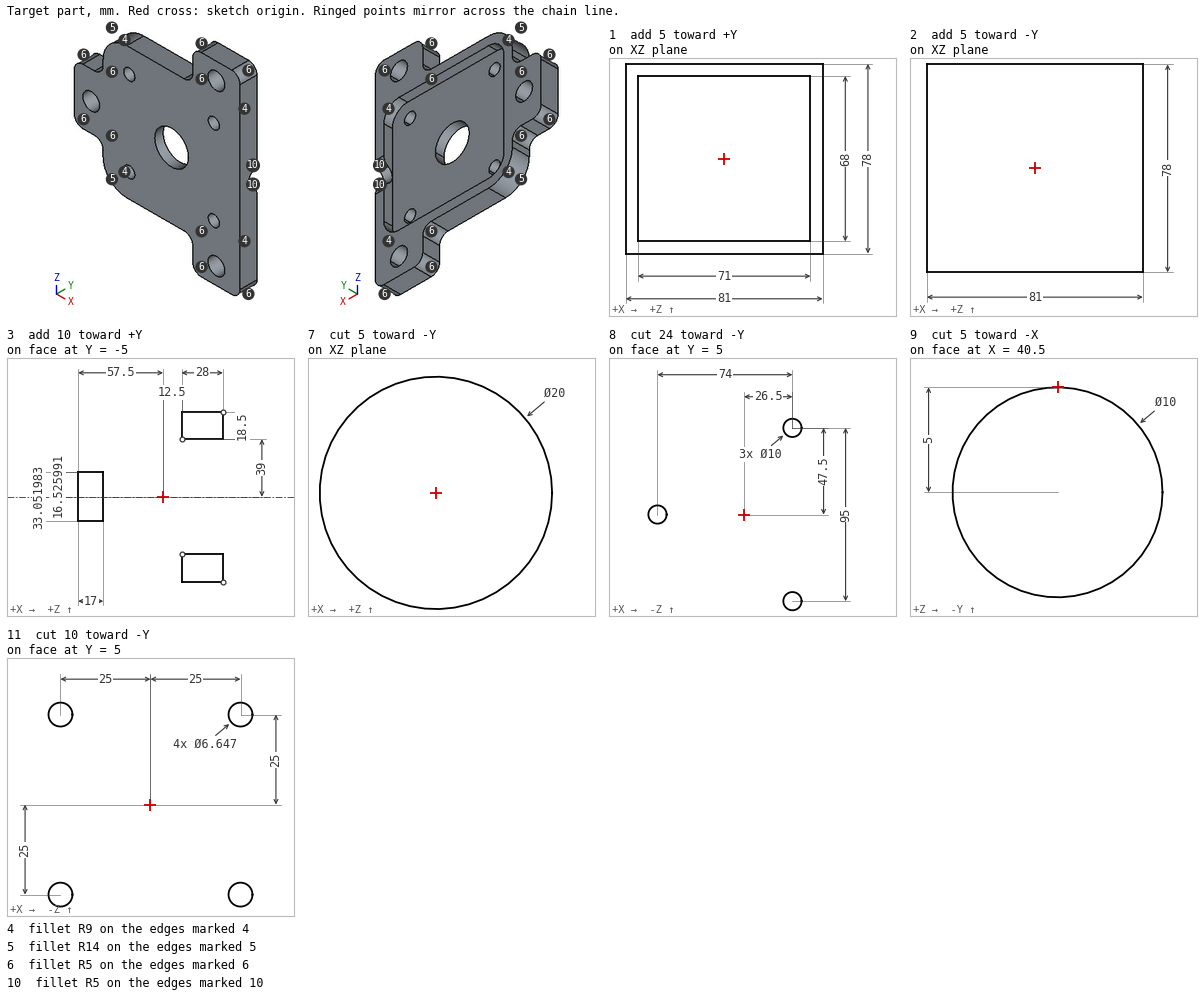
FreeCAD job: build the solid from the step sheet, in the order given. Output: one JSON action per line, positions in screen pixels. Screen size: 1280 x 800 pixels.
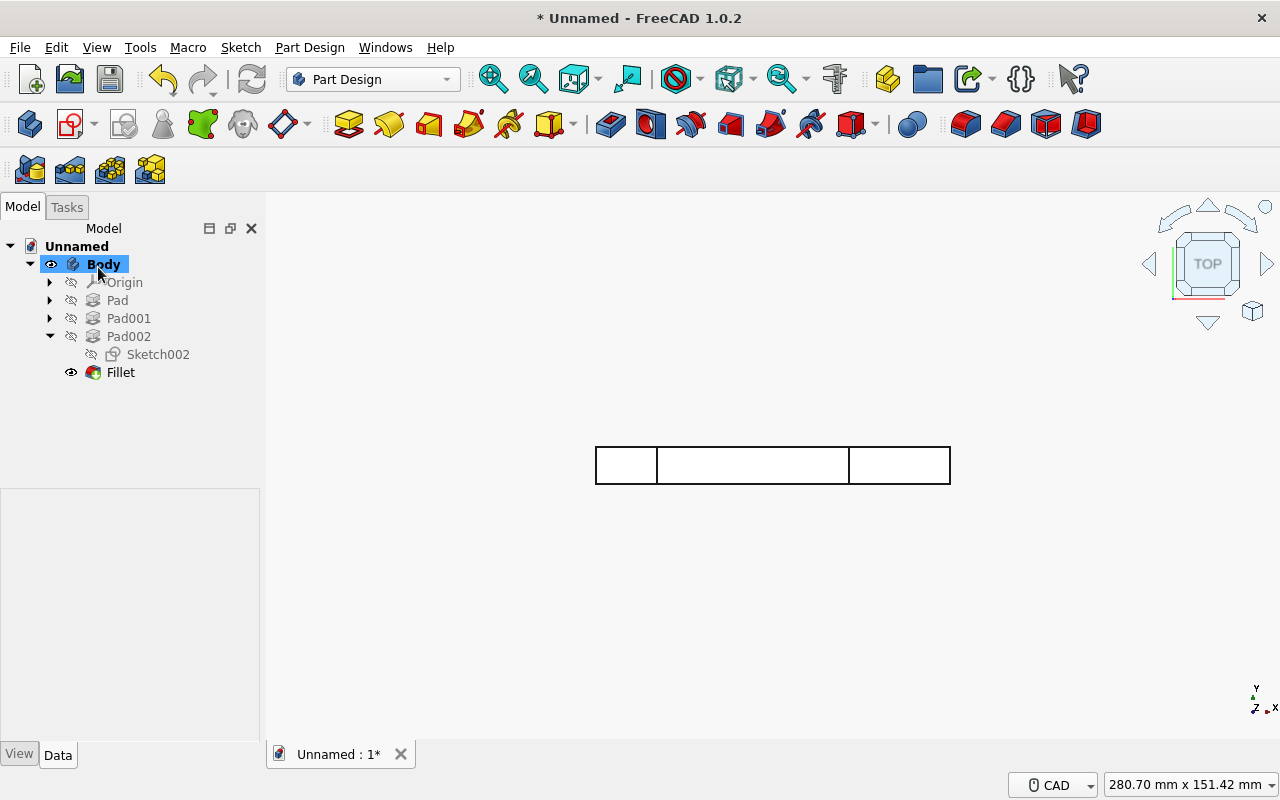
{"action": "key", "text": "v f"}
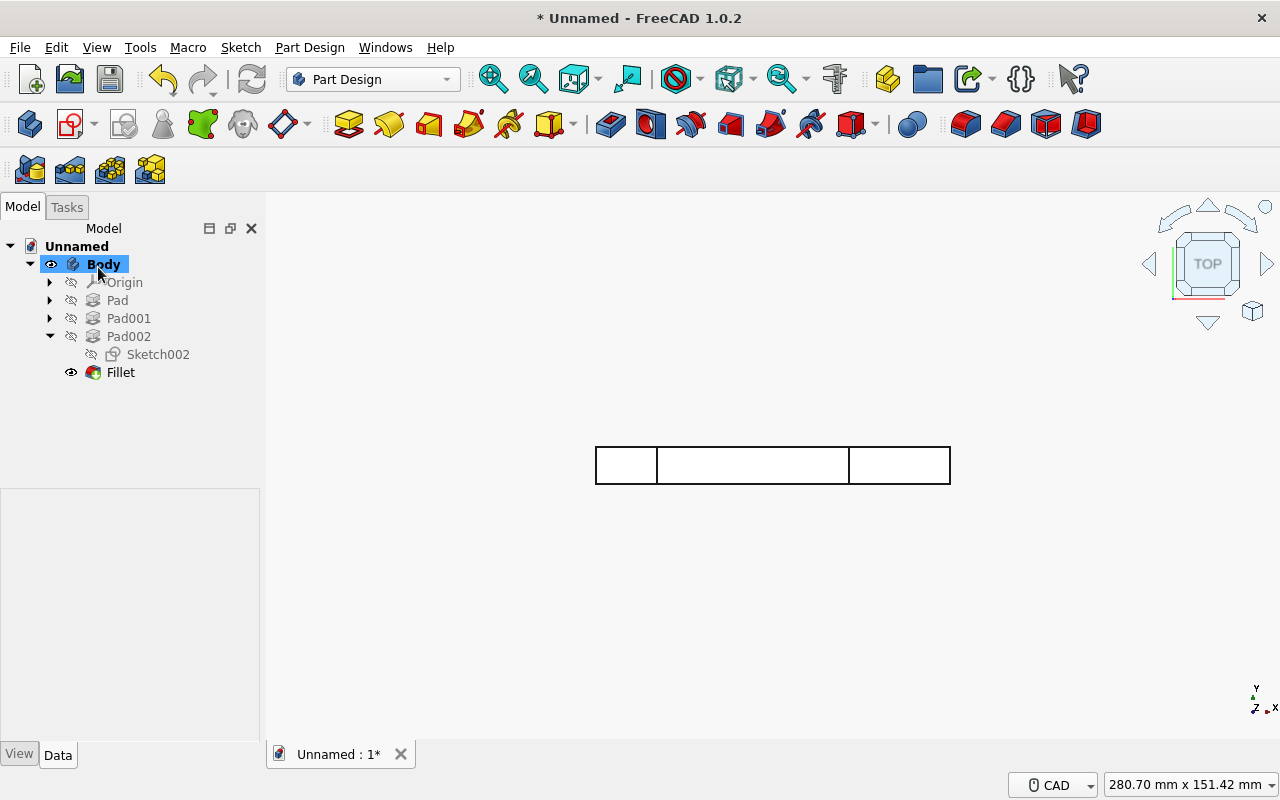
{"action": "left_click", "coordinate": [657, 464]}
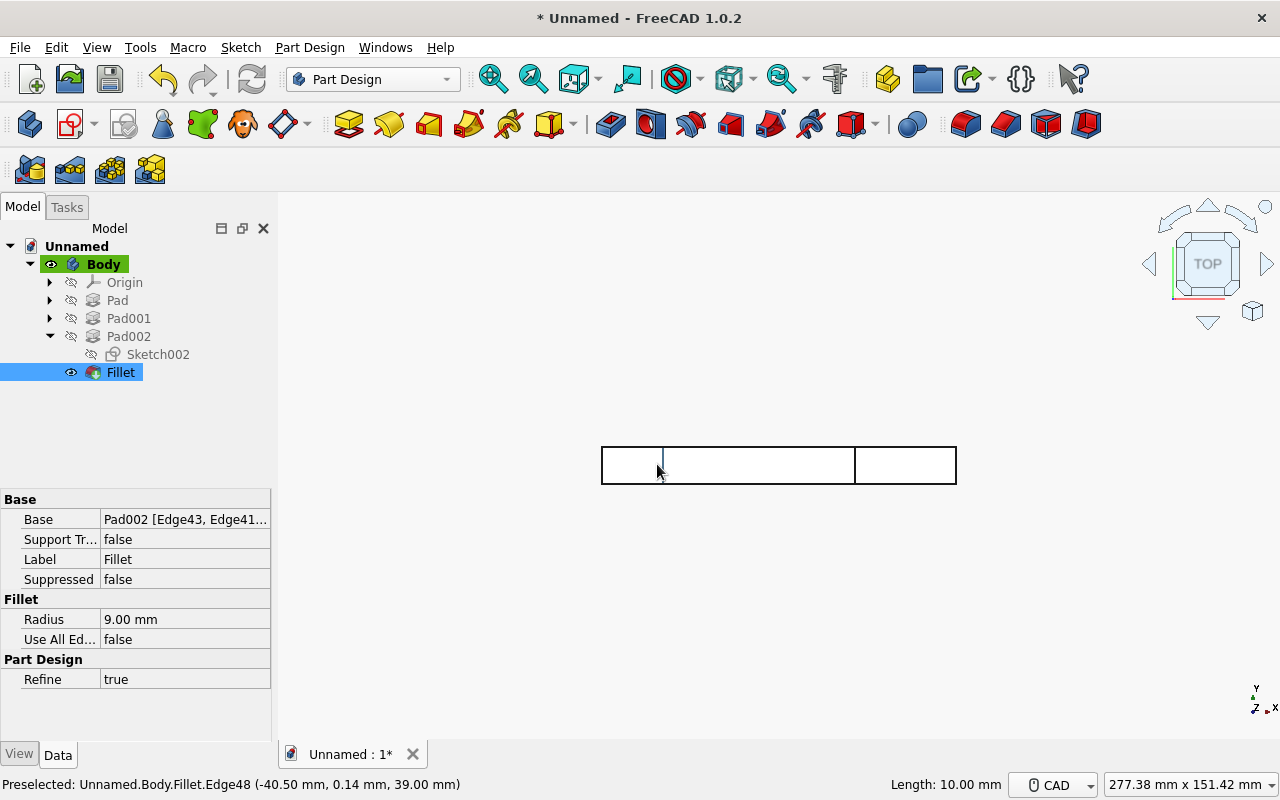
{"action": "key", "text": "0"}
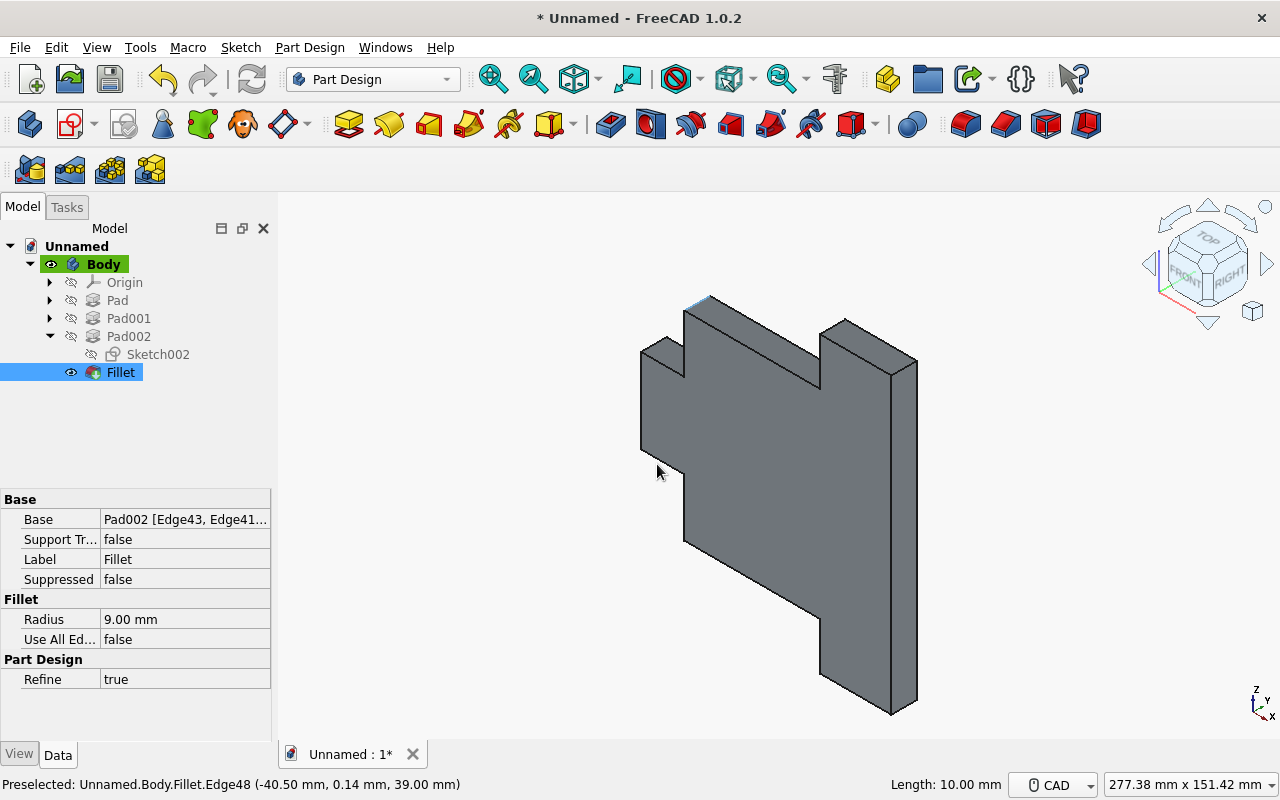
{"action": "key", "text": "1"}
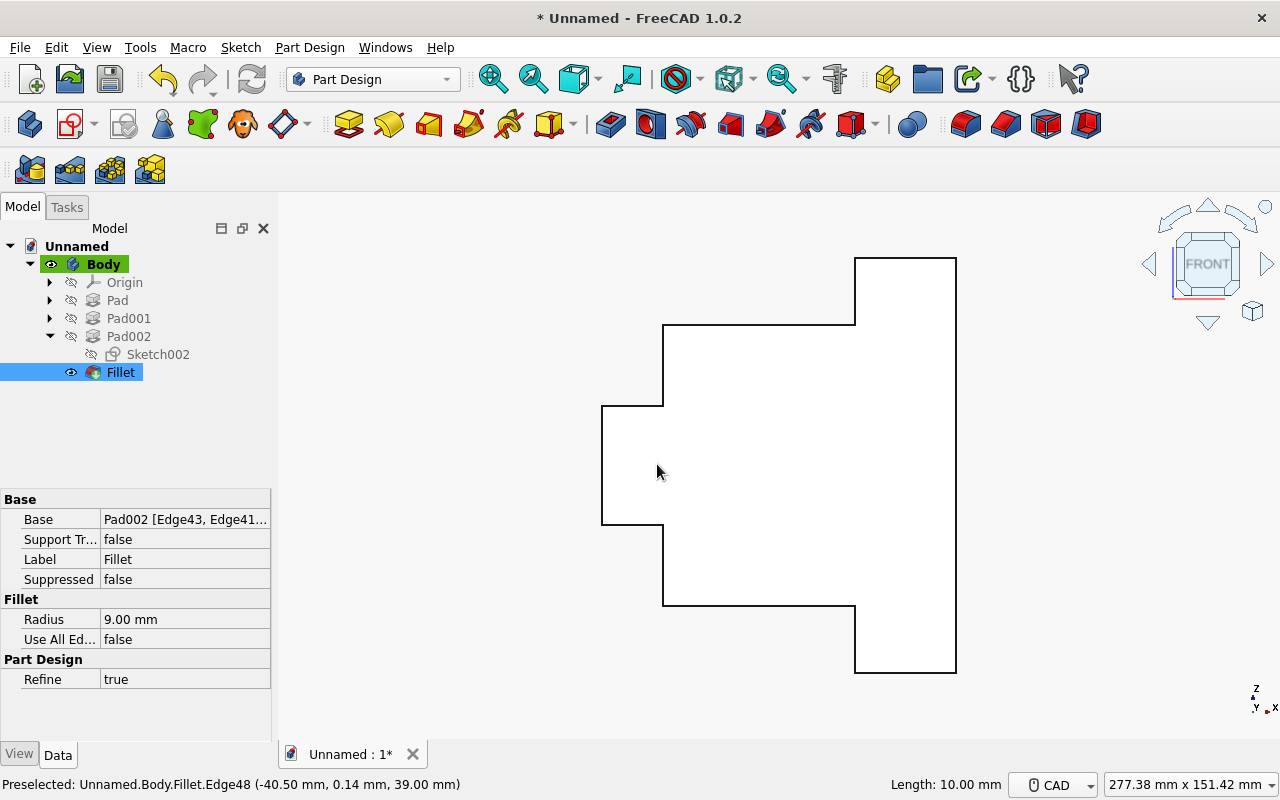
{"action": "key", "text": "3"}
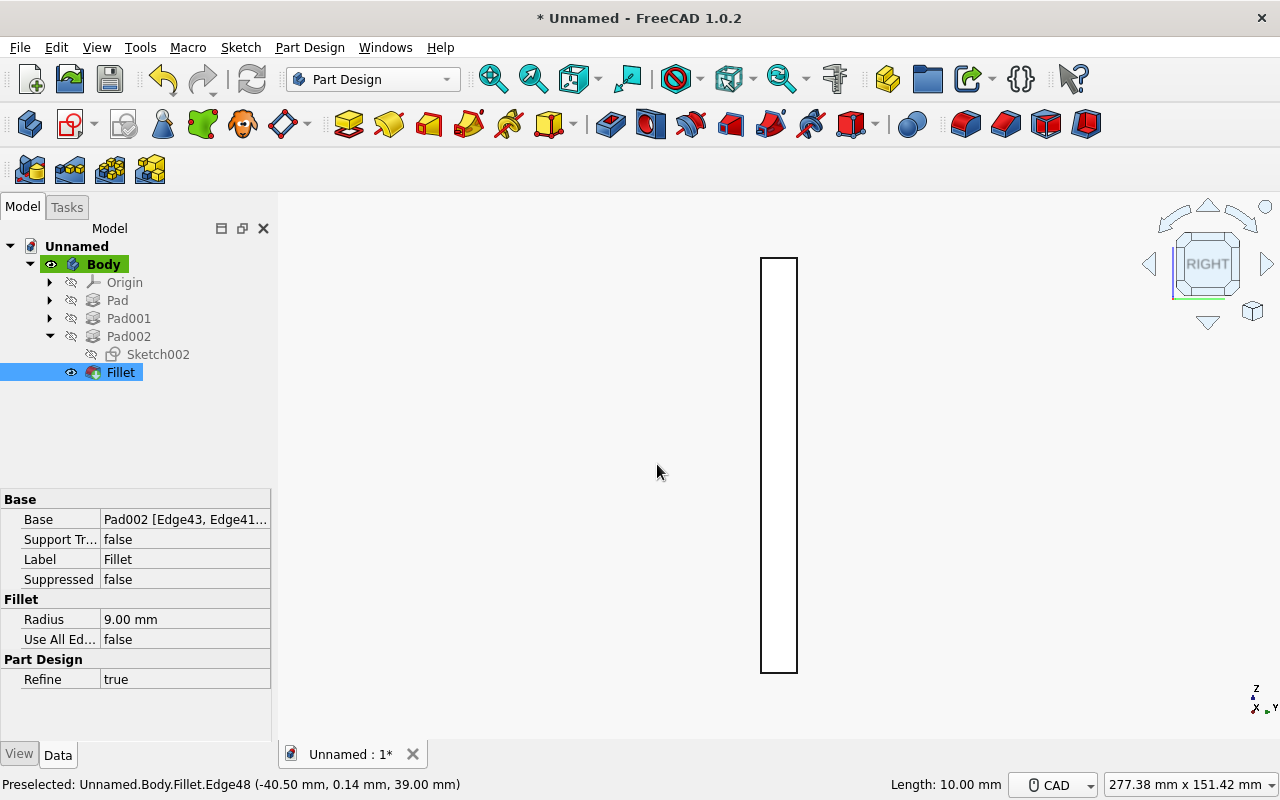
{"action": "key", "text": "5"}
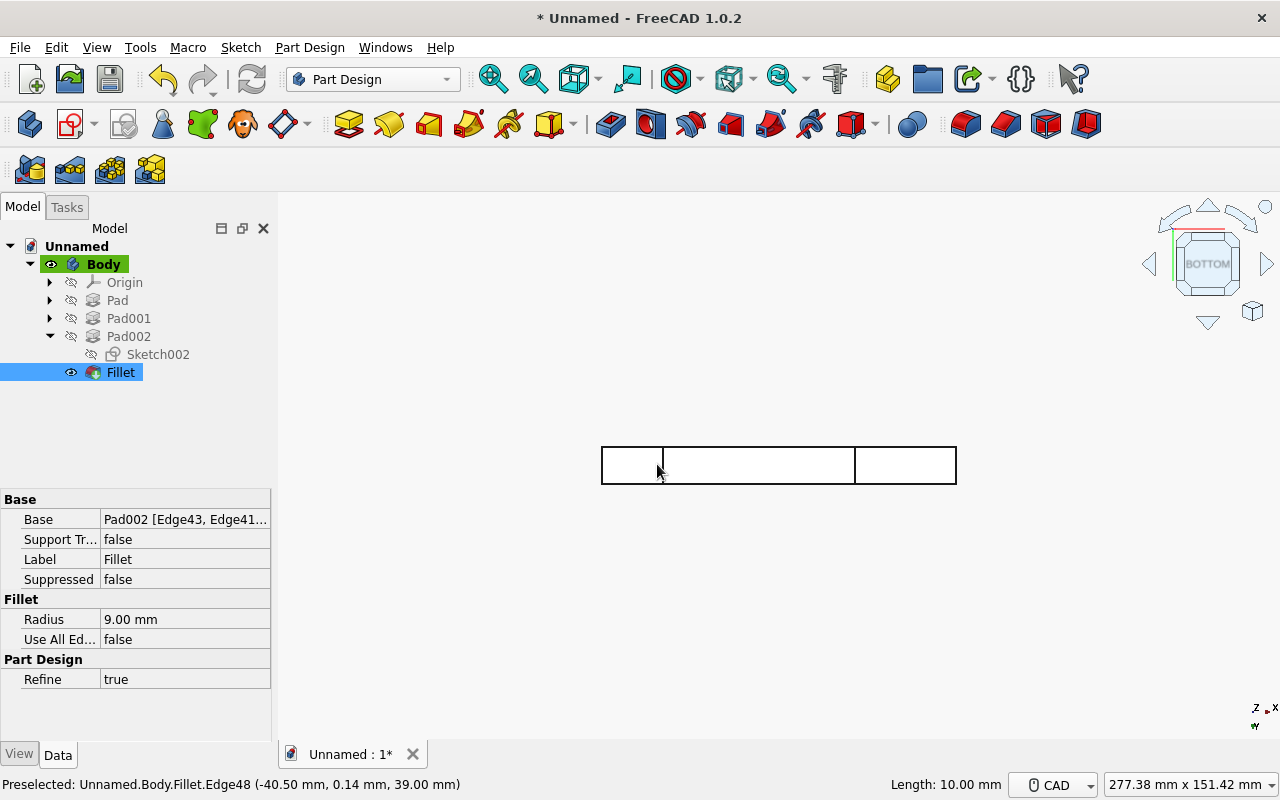
{"action": "key", "text": "v f"}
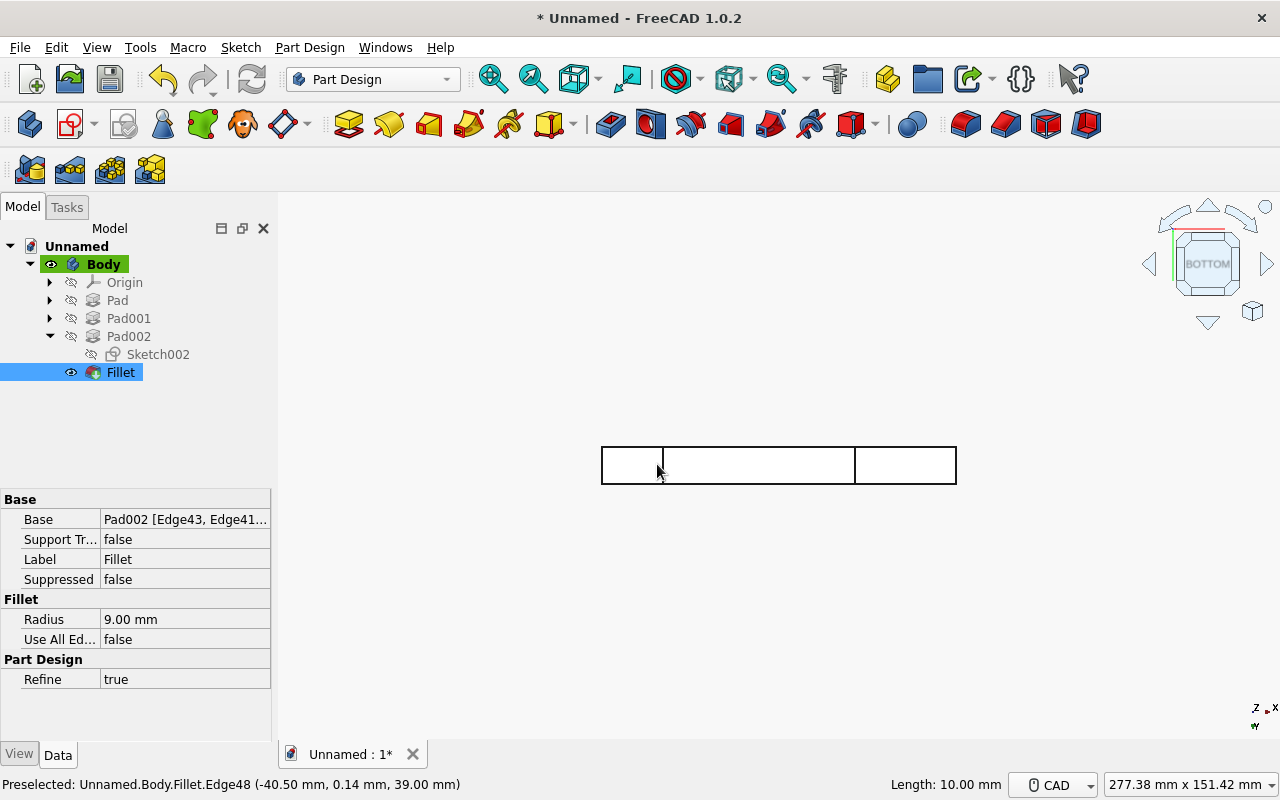
{"action": "left_click", "coordinate": [663, 464], "text": "ctrl"}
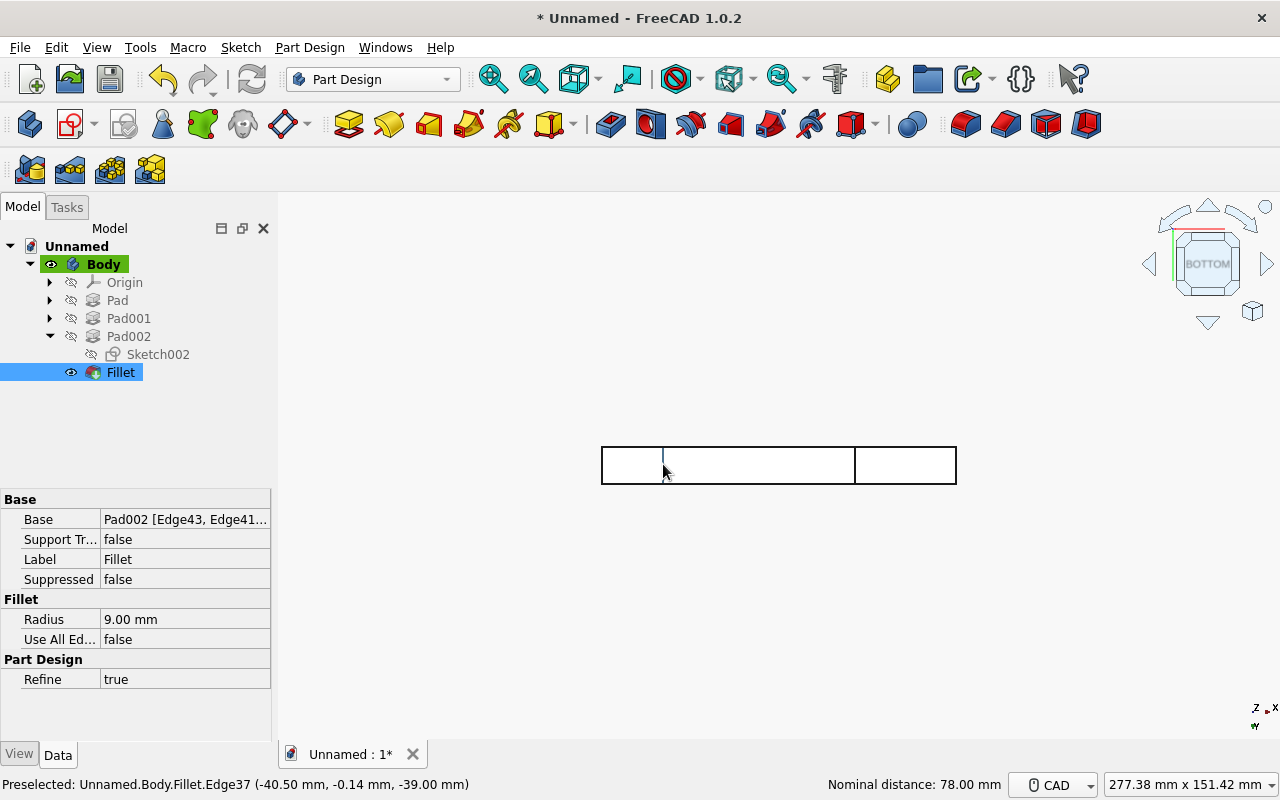
{"action": "left_click", "coordinate": [966, 124]}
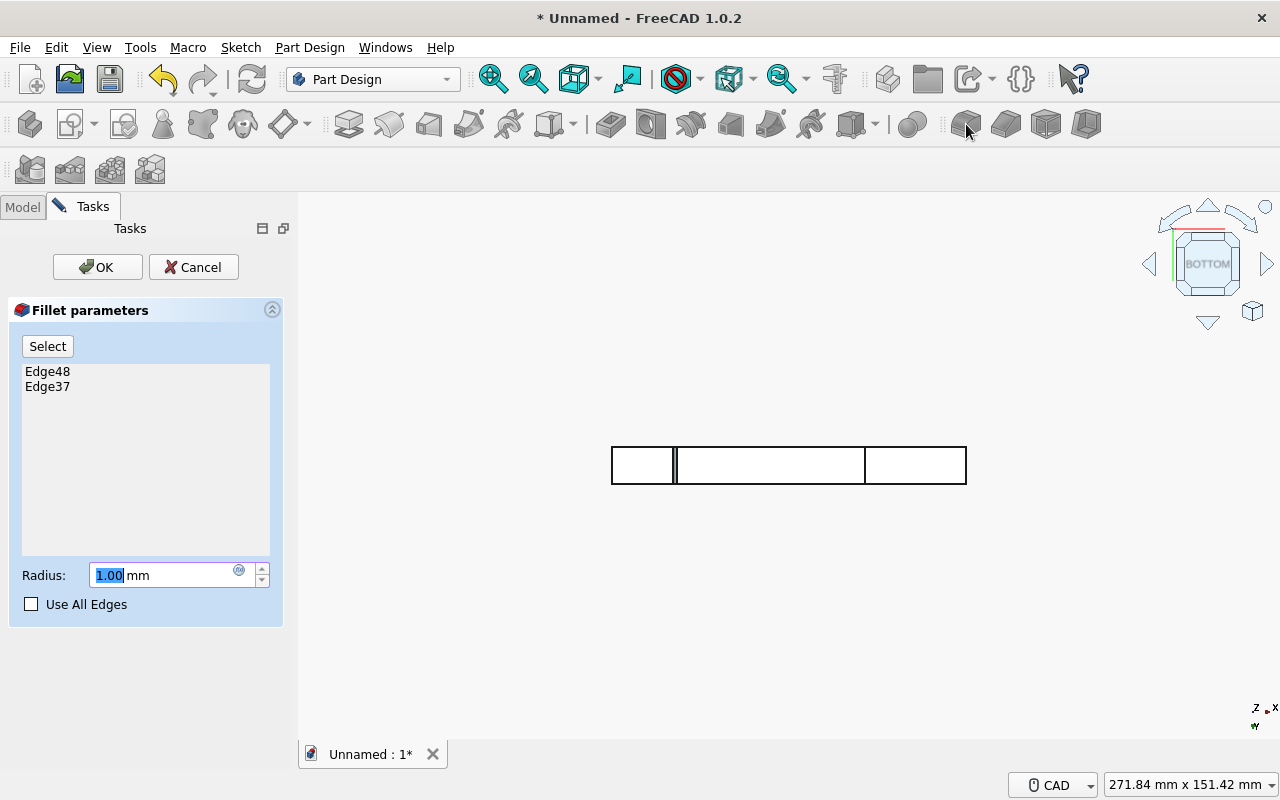
{"action": "type", "text": "14"}
{"action": "key", "text": "Tab"}